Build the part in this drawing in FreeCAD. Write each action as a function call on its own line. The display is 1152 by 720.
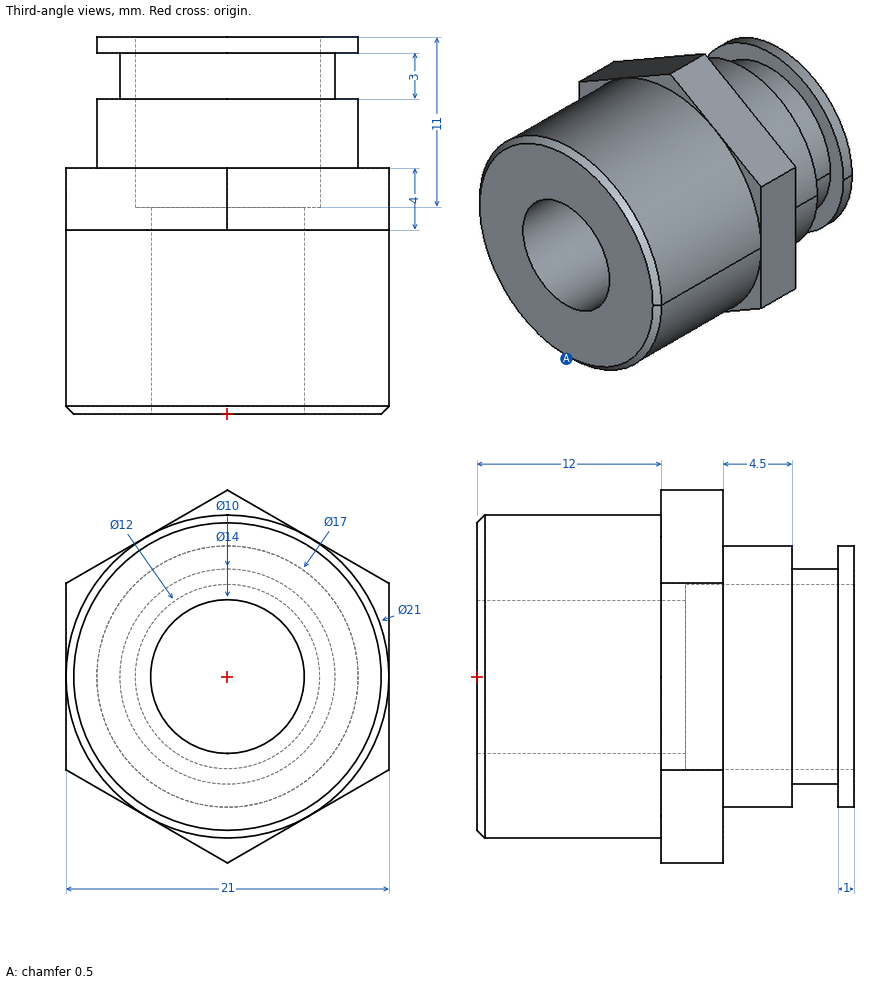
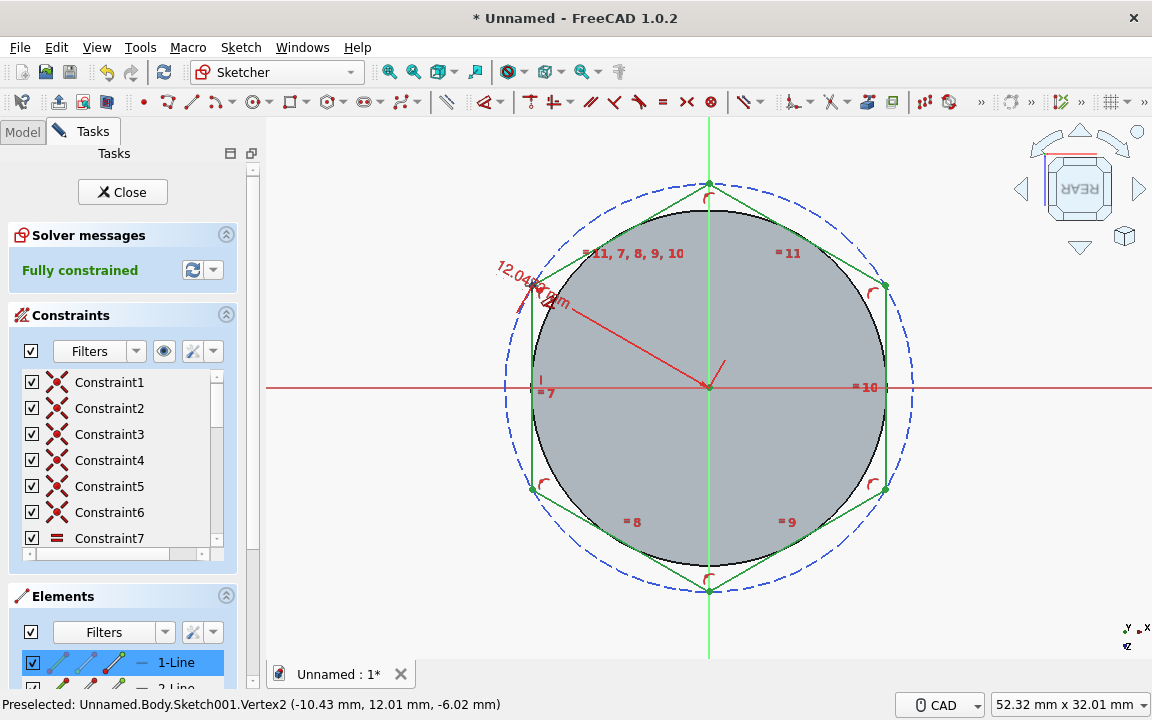
click(886, 490)
click(628, 524)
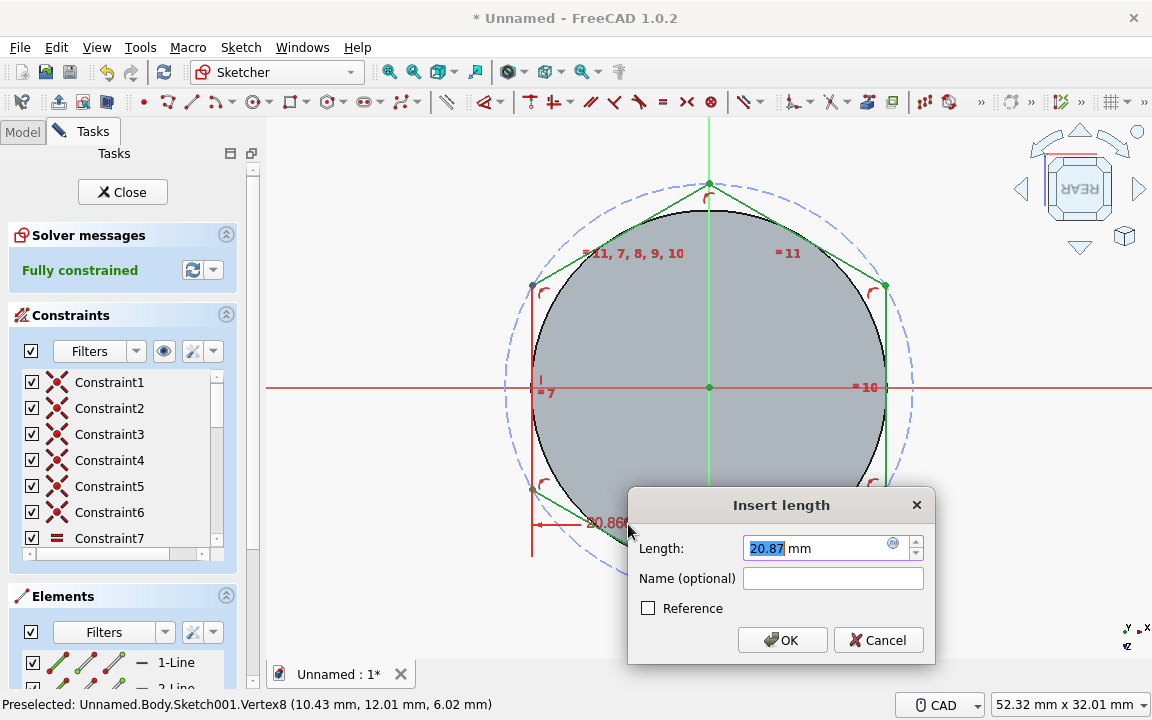
text(21)
key(Return)
key(Escape)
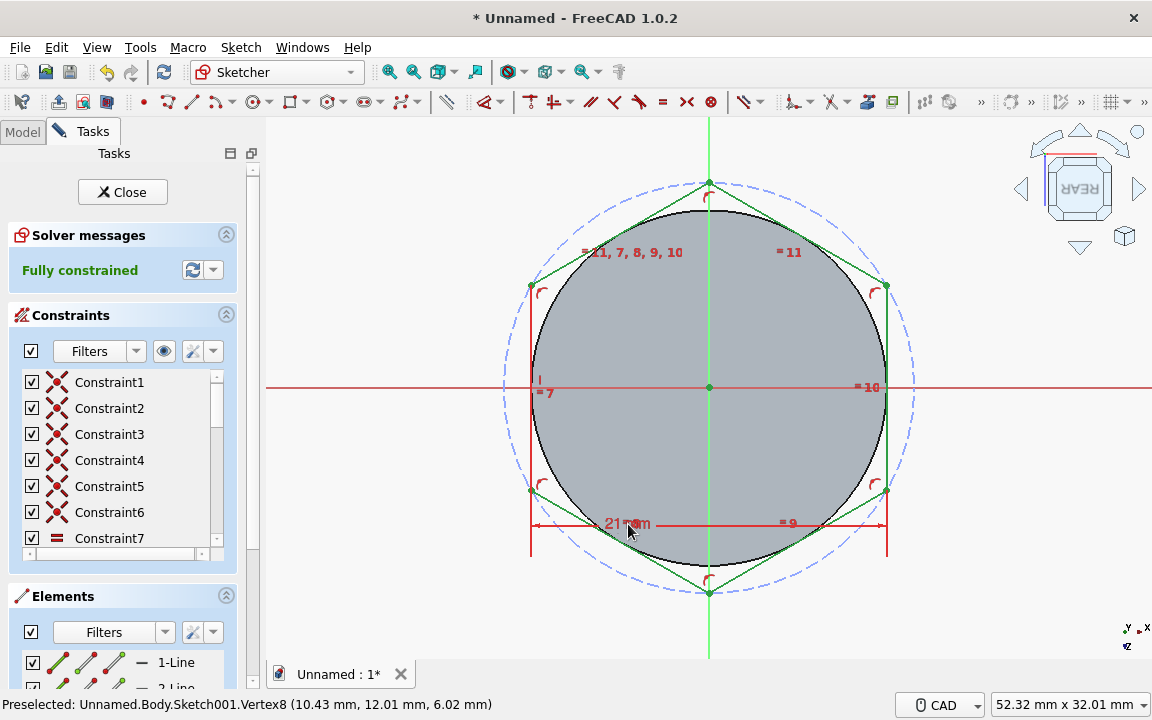
click(123, 192)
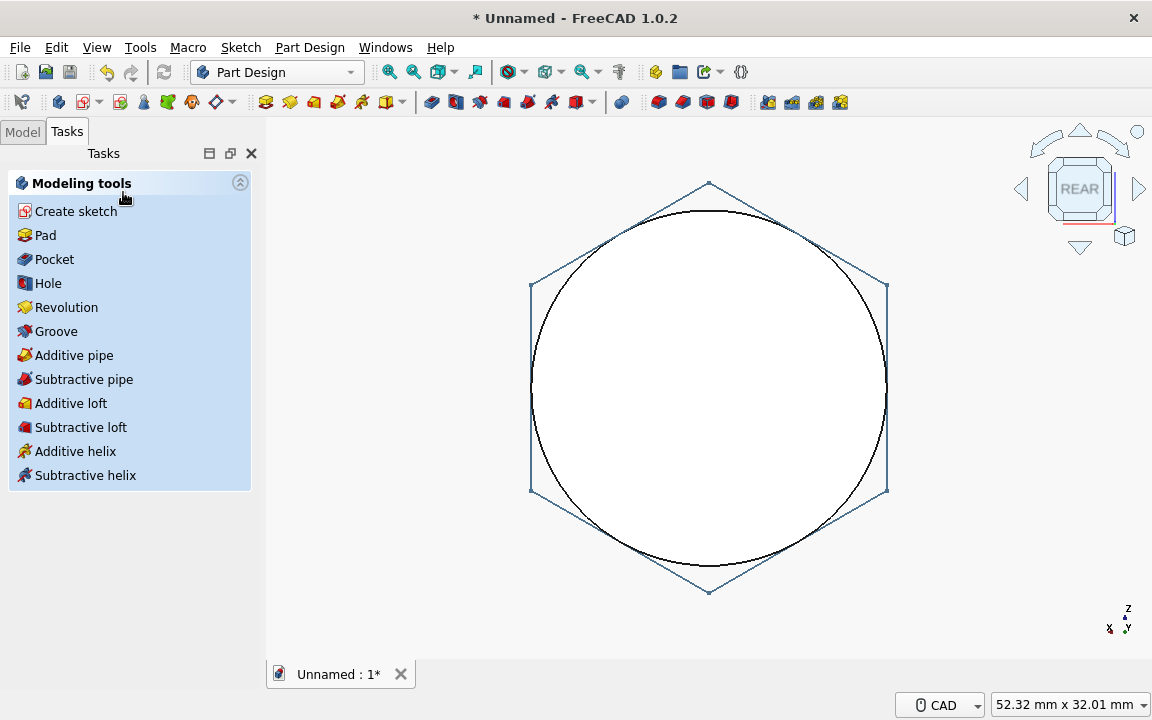
click(266, 102)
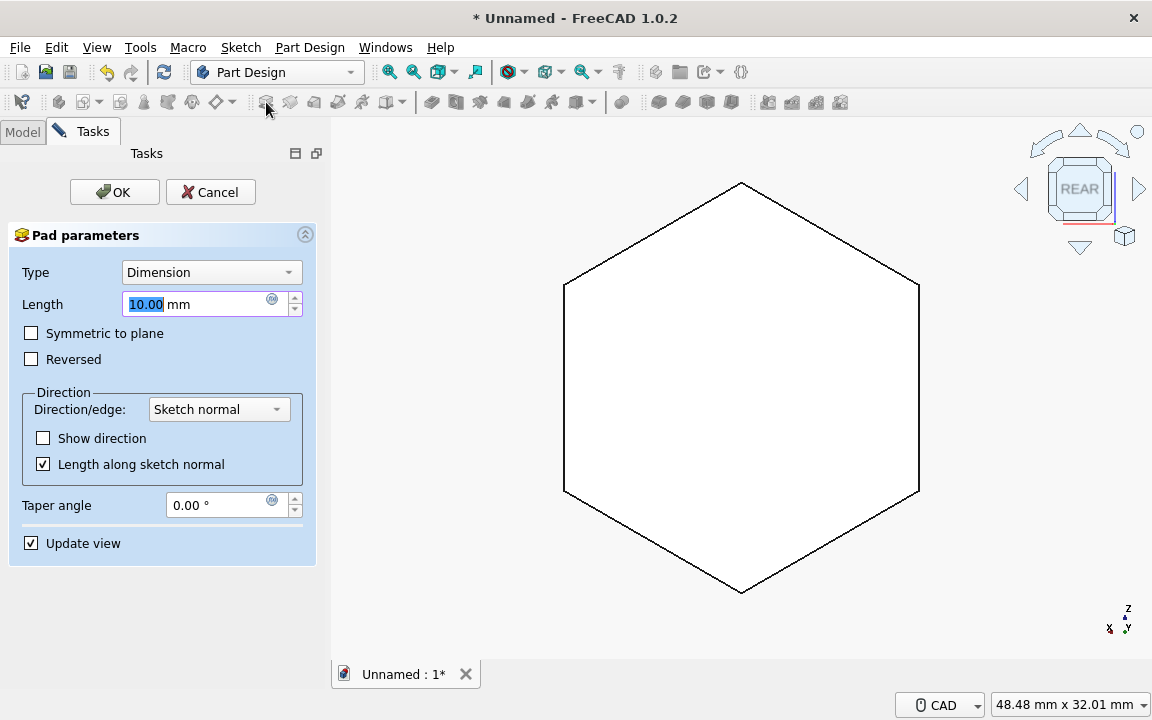
text(4)
key(Tab)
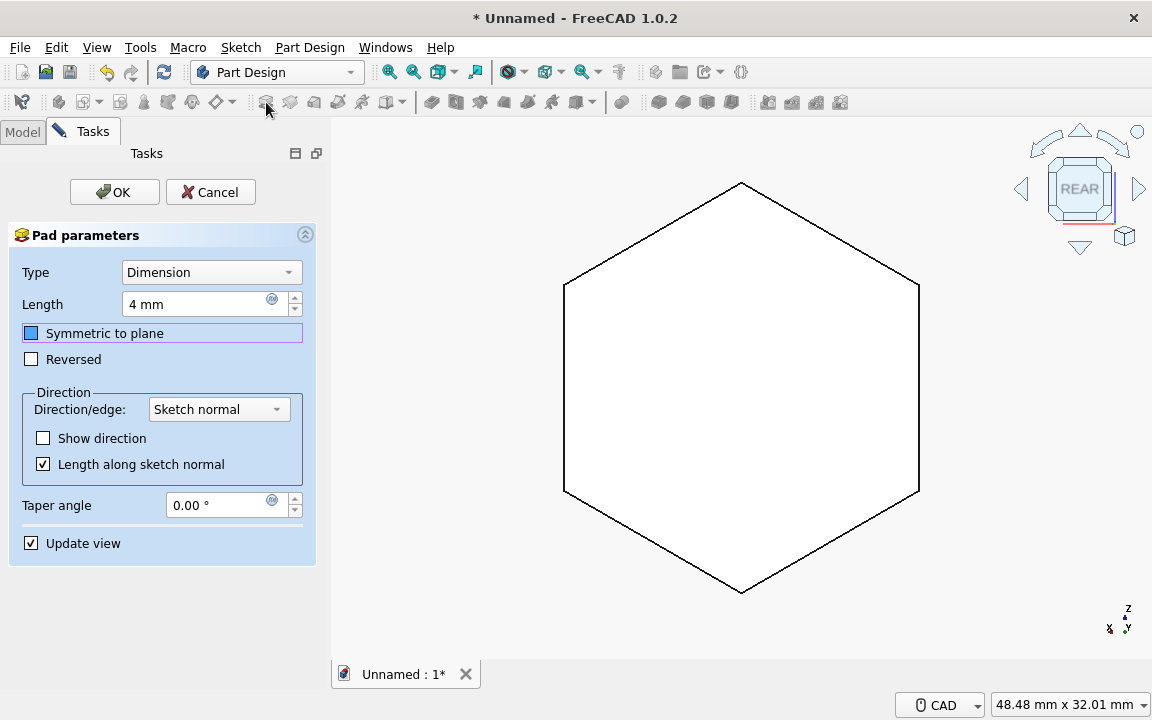
click(115, 192)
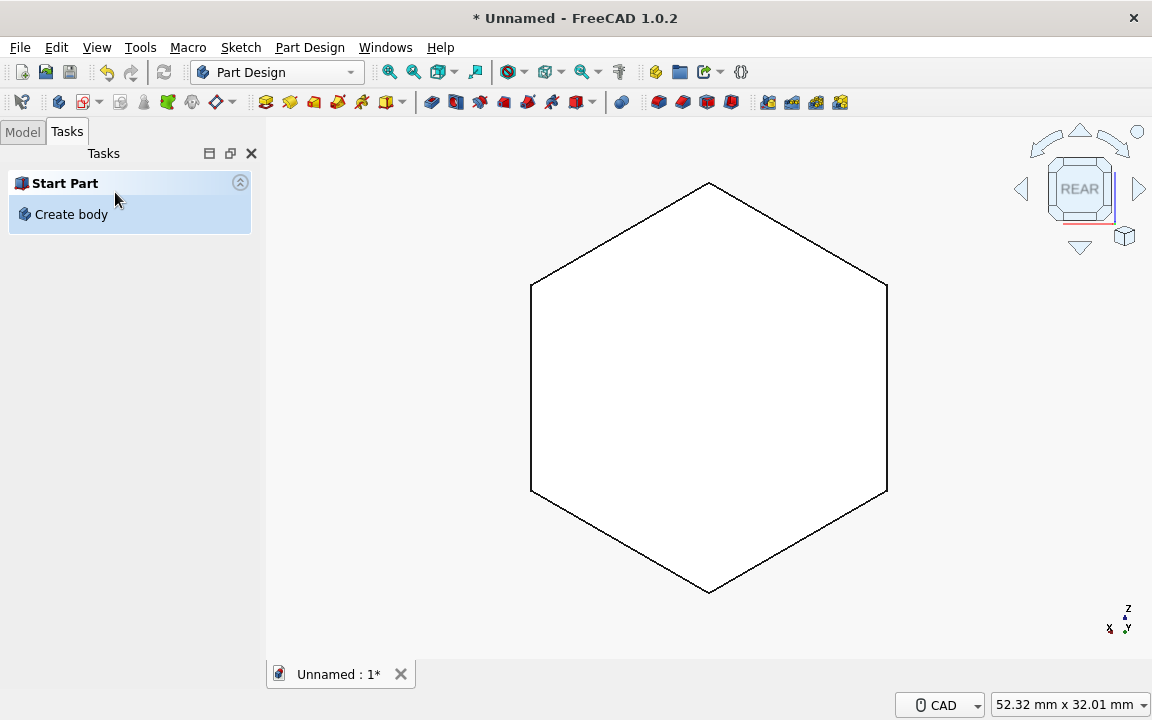
click(709, 387)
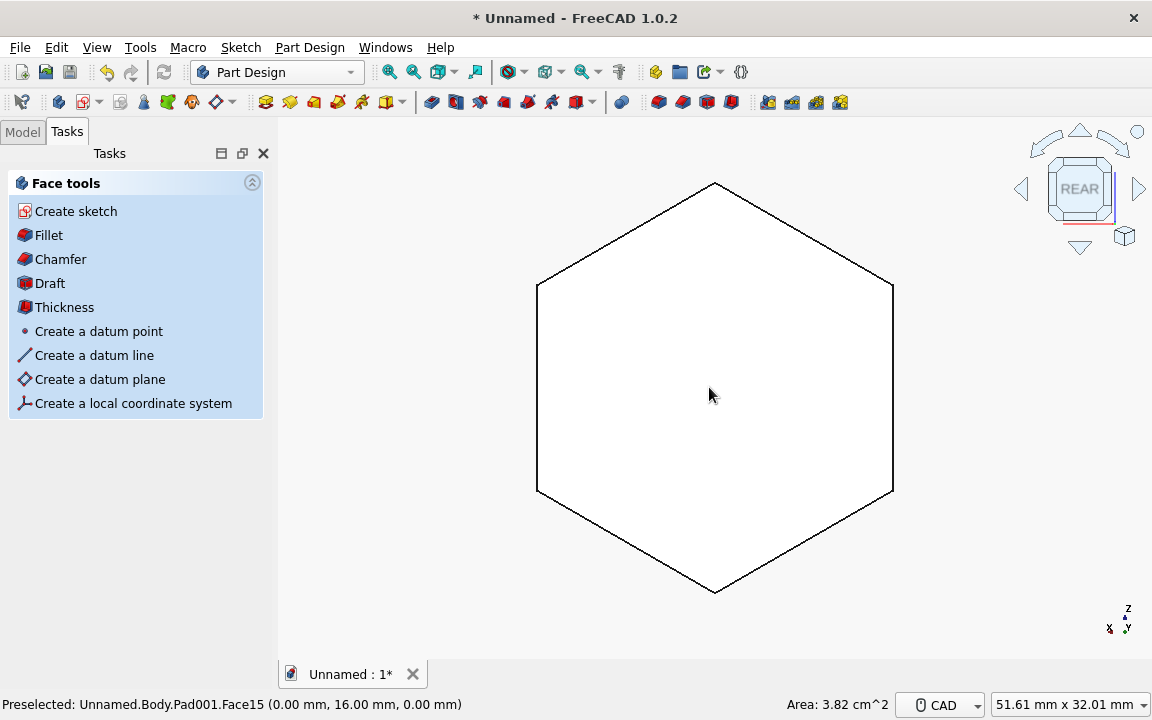
click(84, 102)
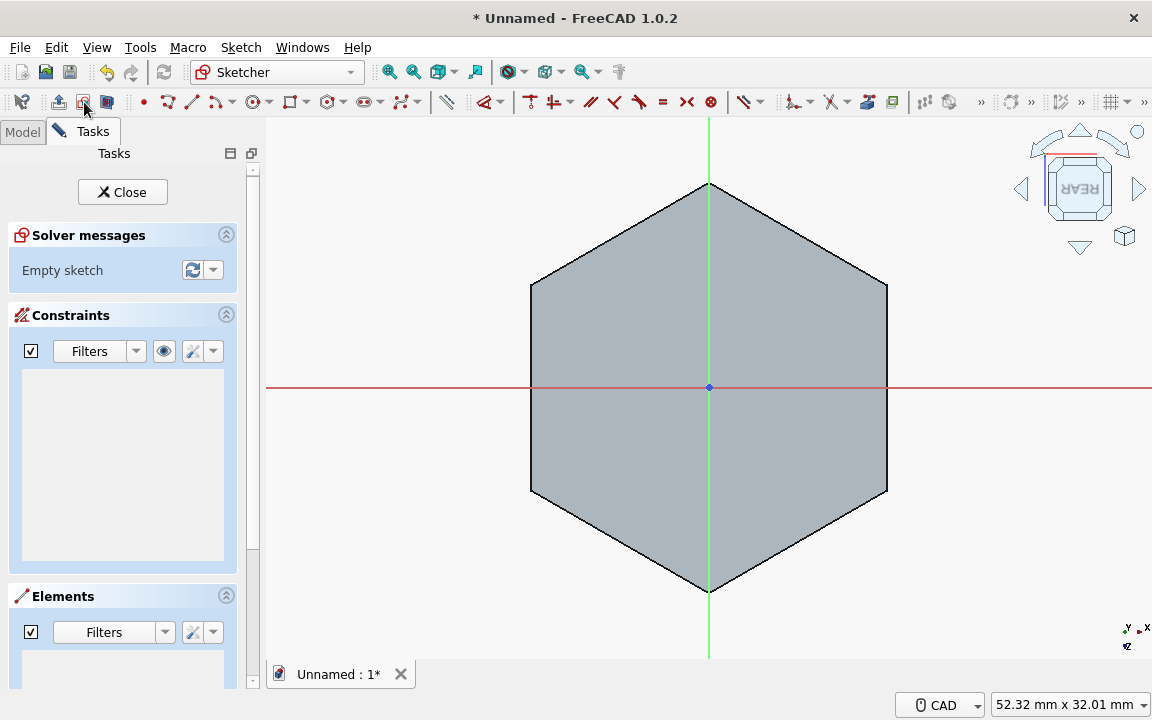
click(254, 102)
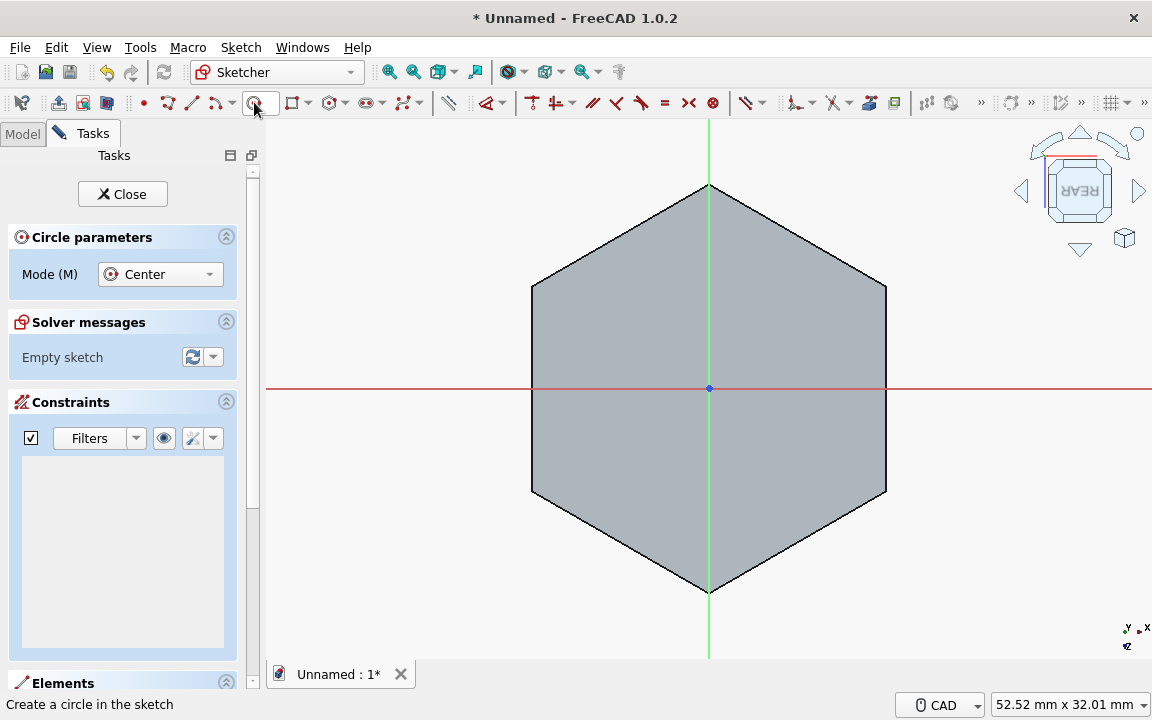
click(709, 389)
move(810, 288)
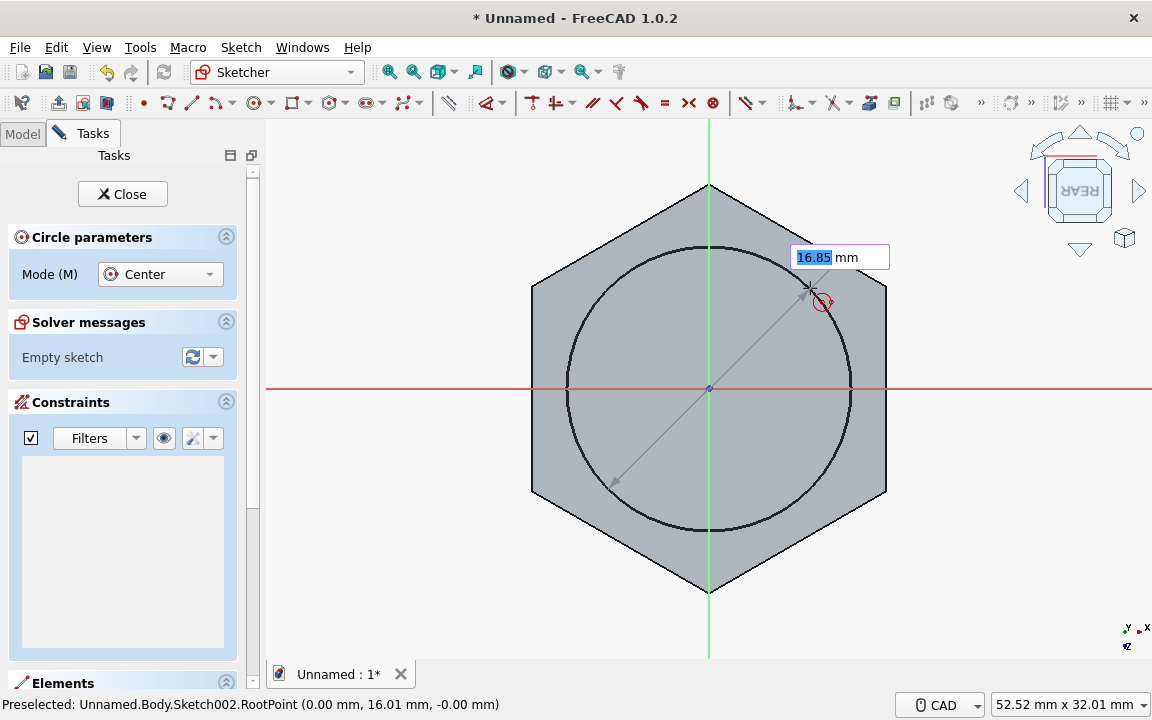
text(17)
key(Return)
key(Escape)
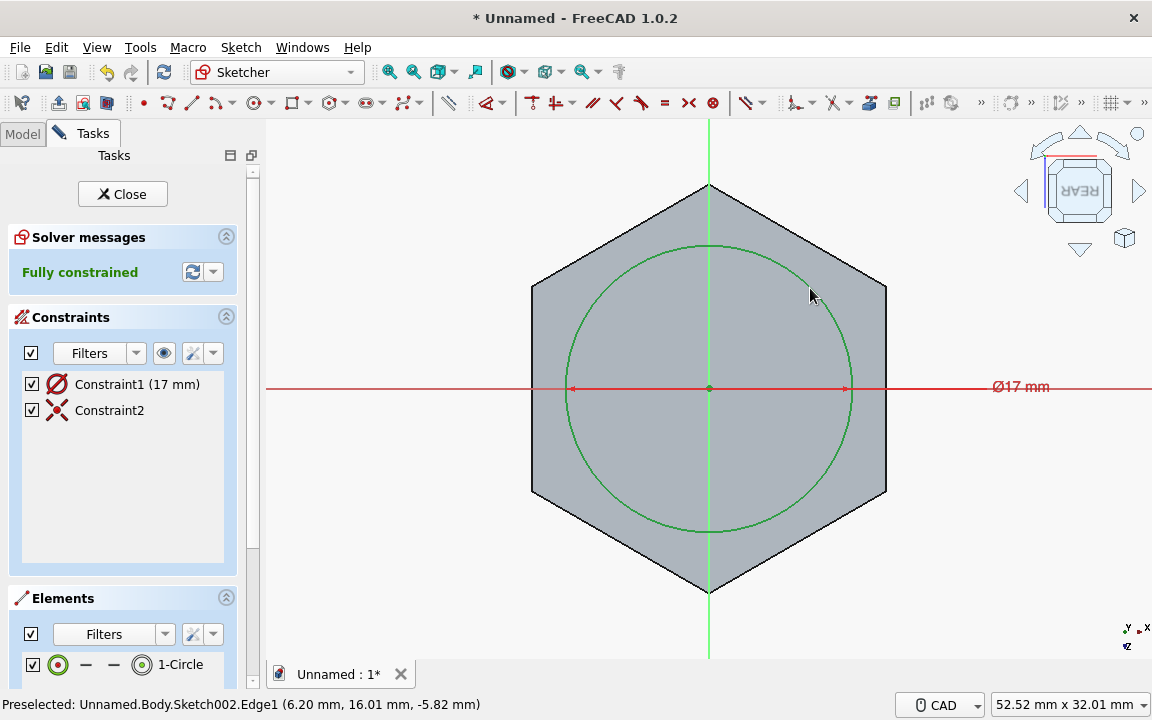
click(123, 194)